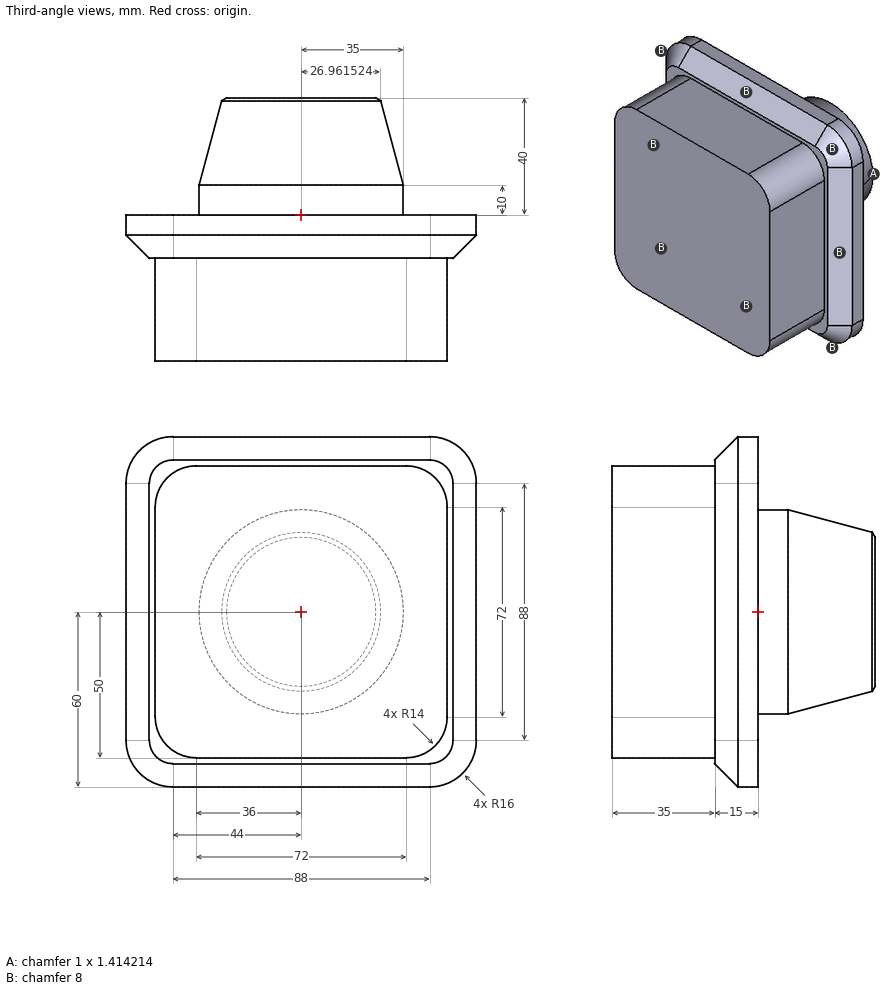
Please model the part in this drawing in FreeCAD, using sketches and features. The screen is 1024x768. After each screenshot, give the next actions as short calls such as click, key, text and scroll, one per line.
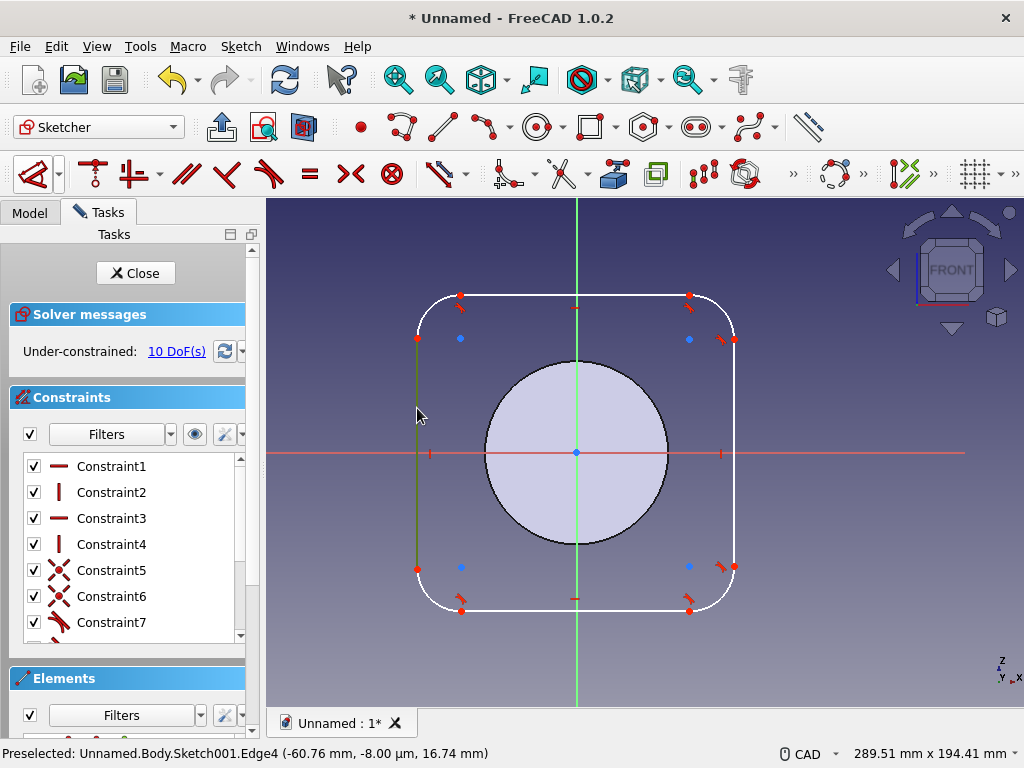
click(441, 300)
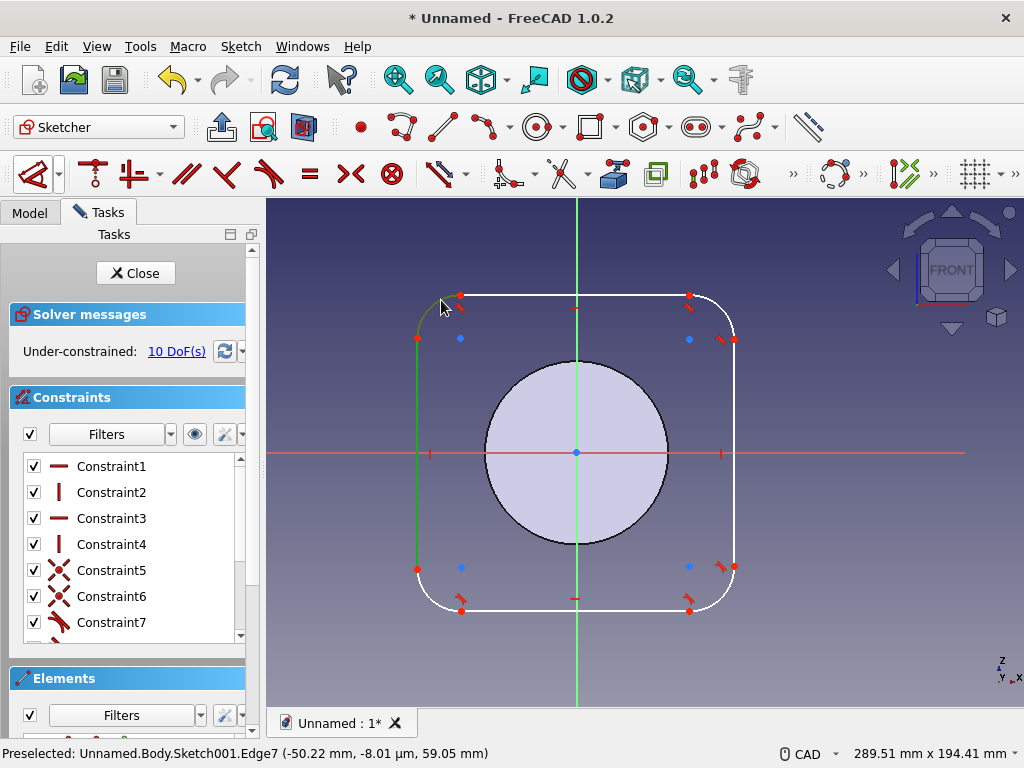
key(t)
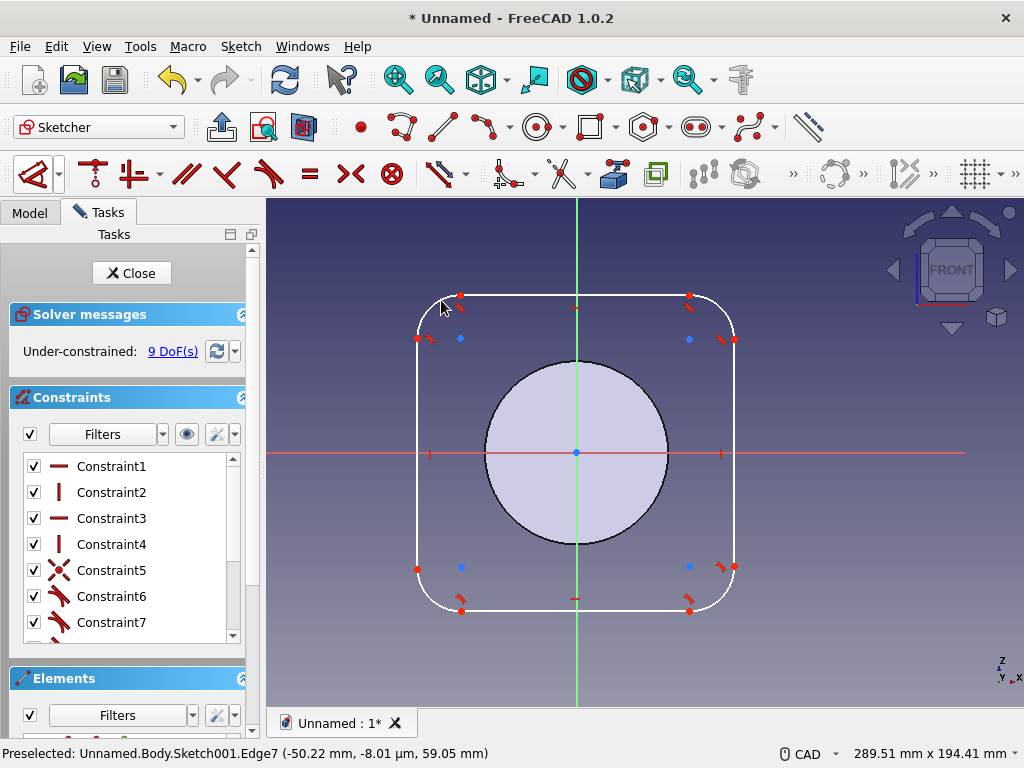
click(417, 408)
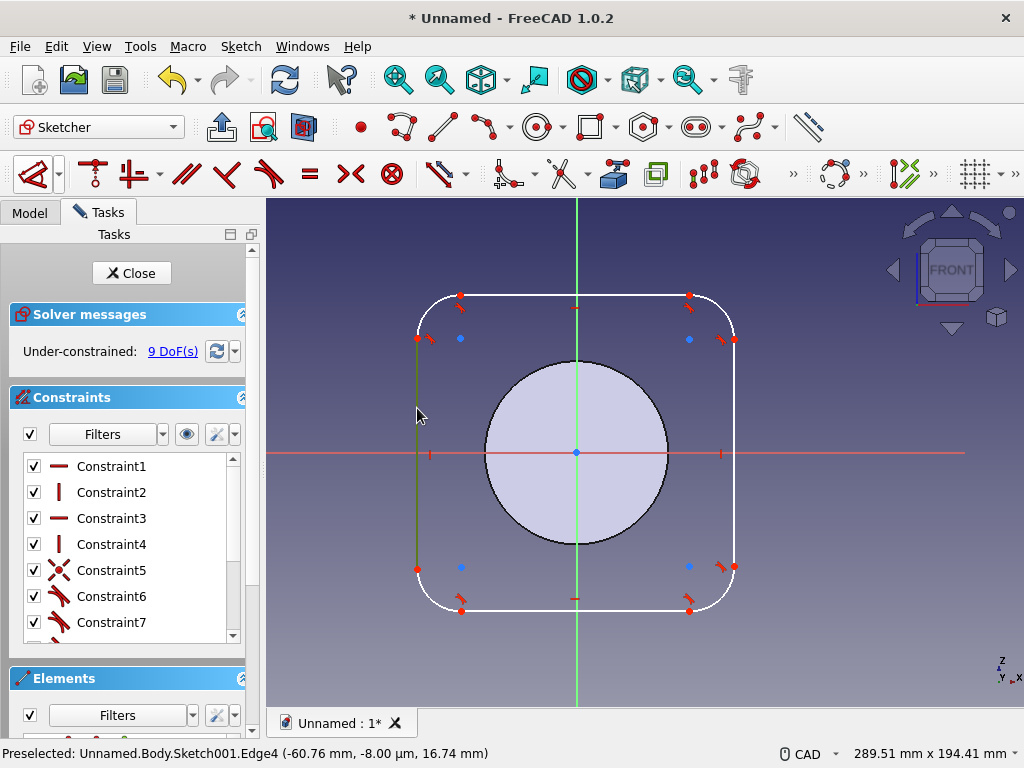
click(423, 589)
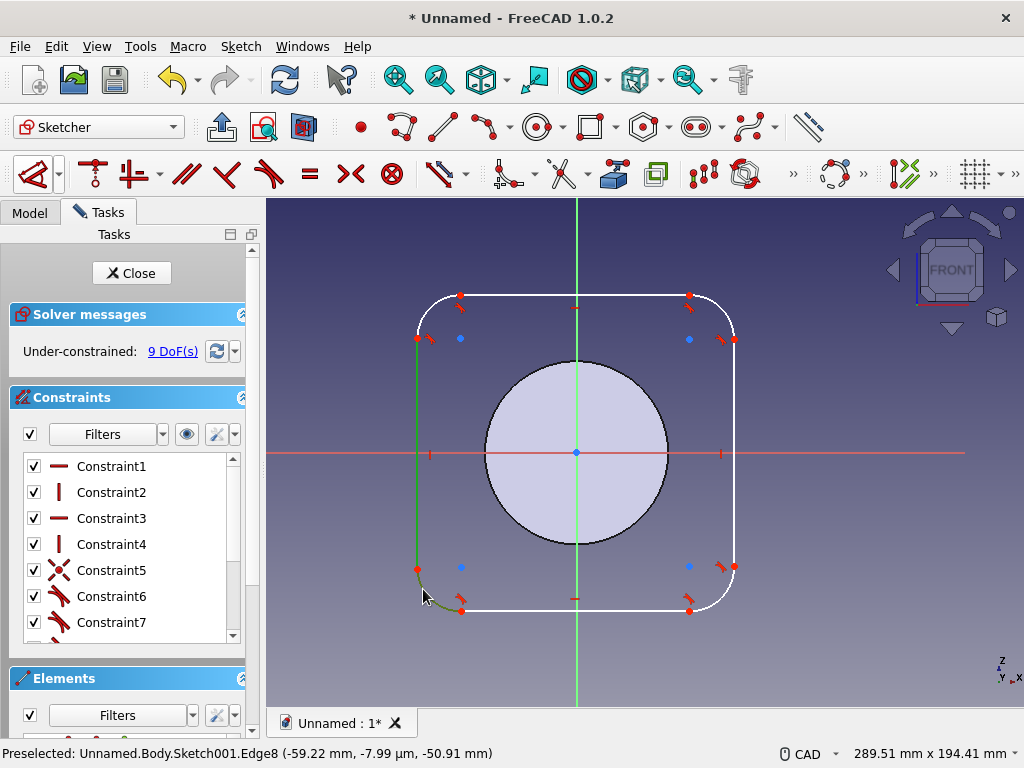
key(t)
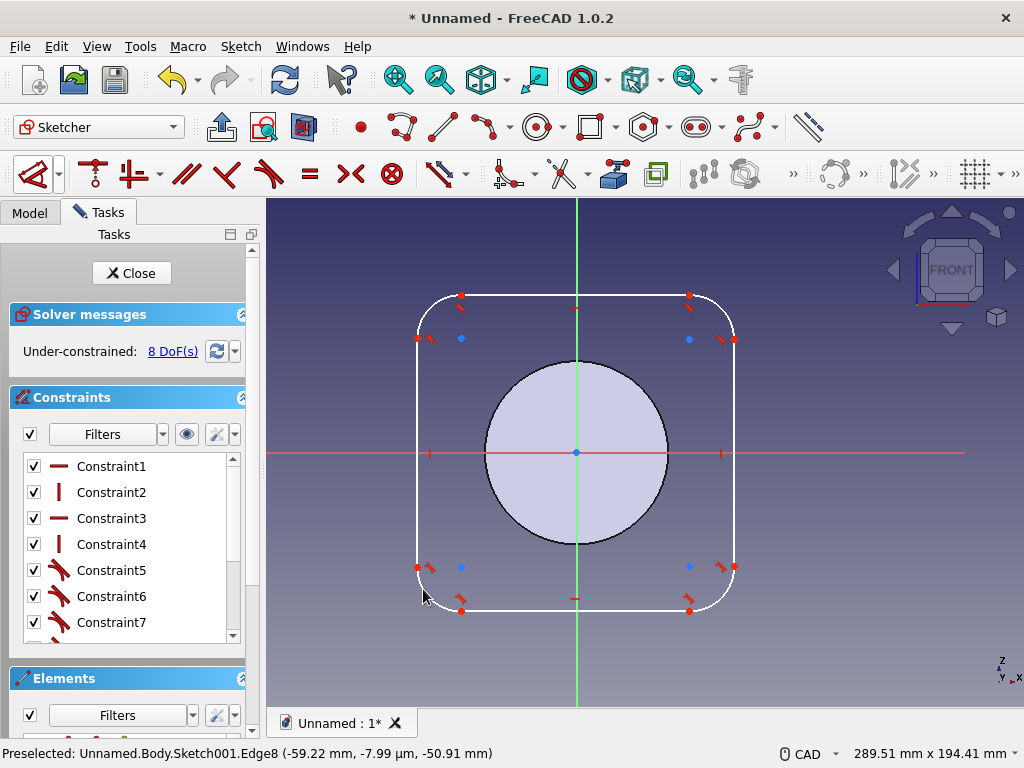
click(710, 607)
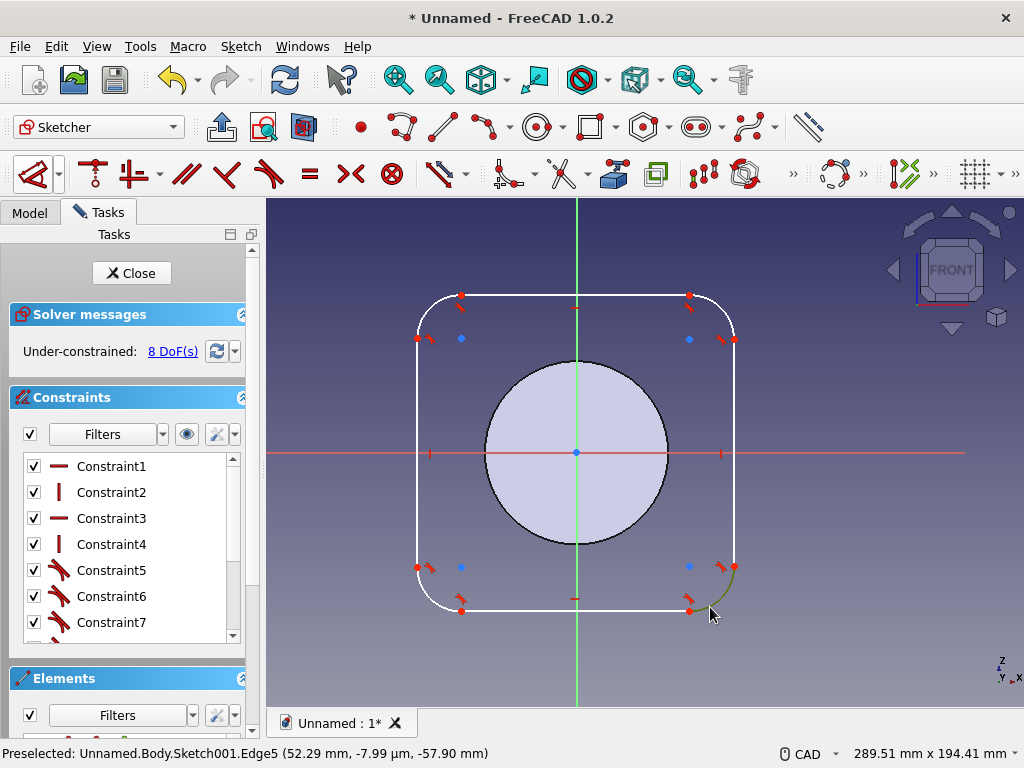
click(729, 319)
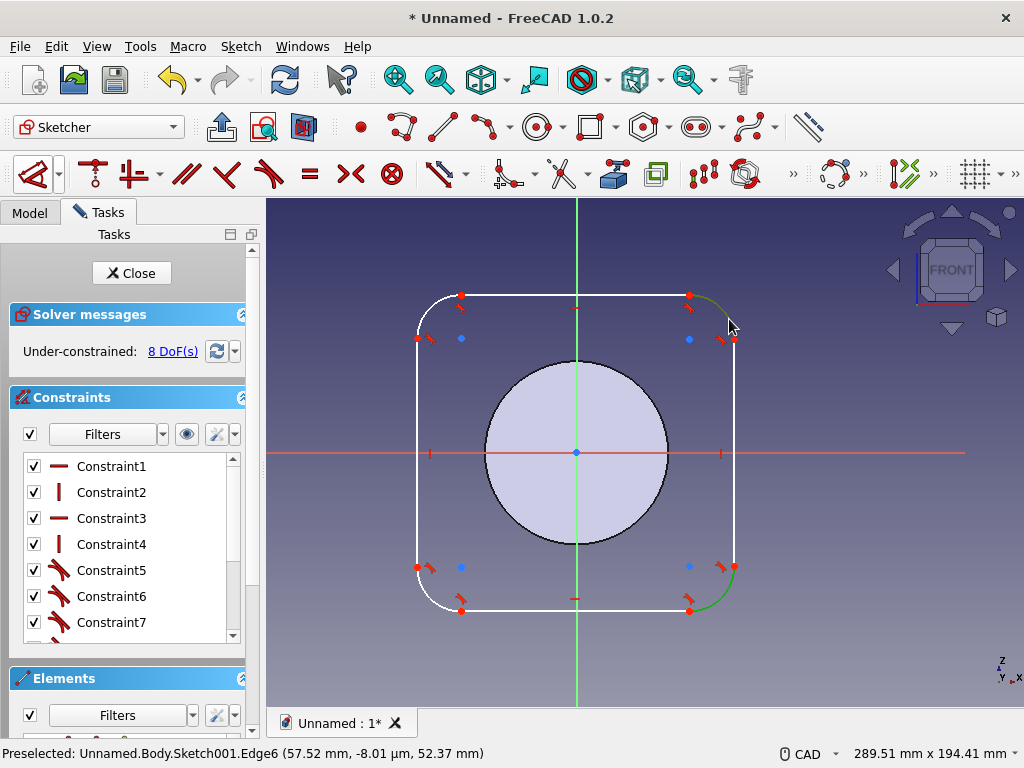
click(441, 300)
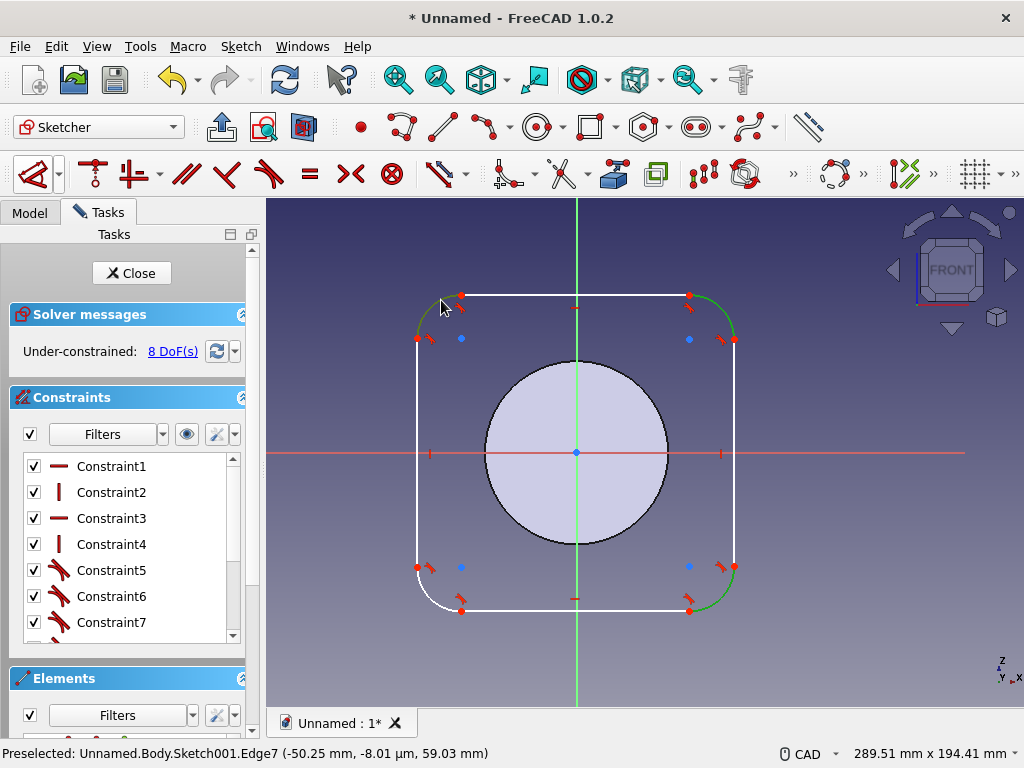
click(422, 588)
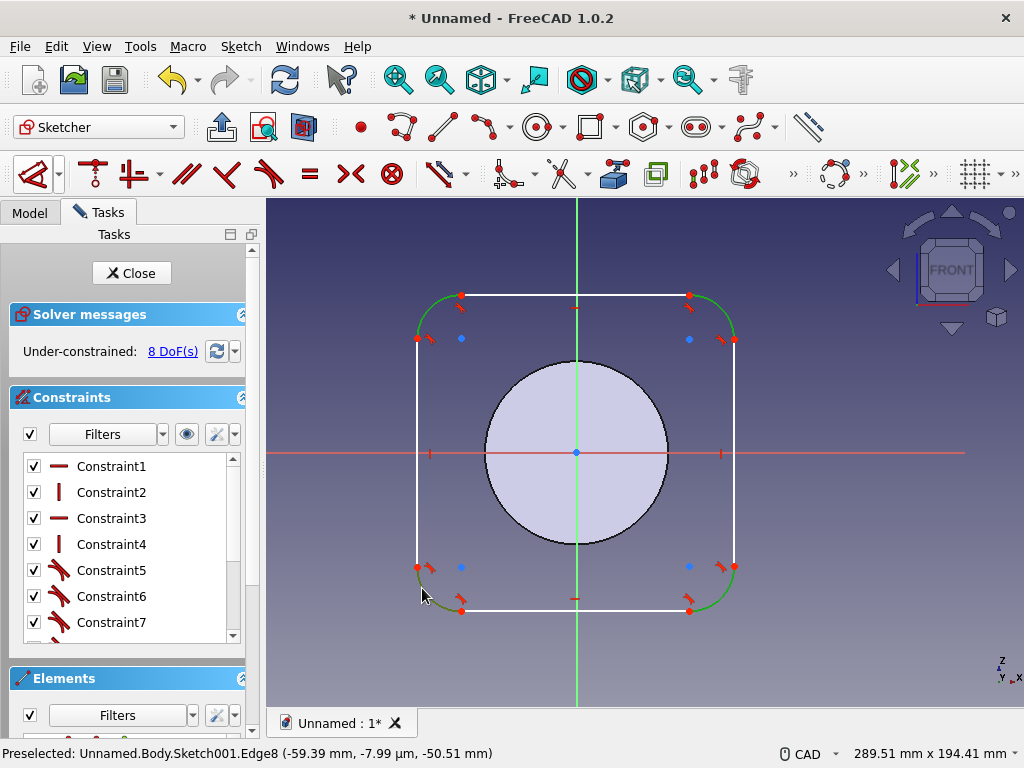
click(310, 174)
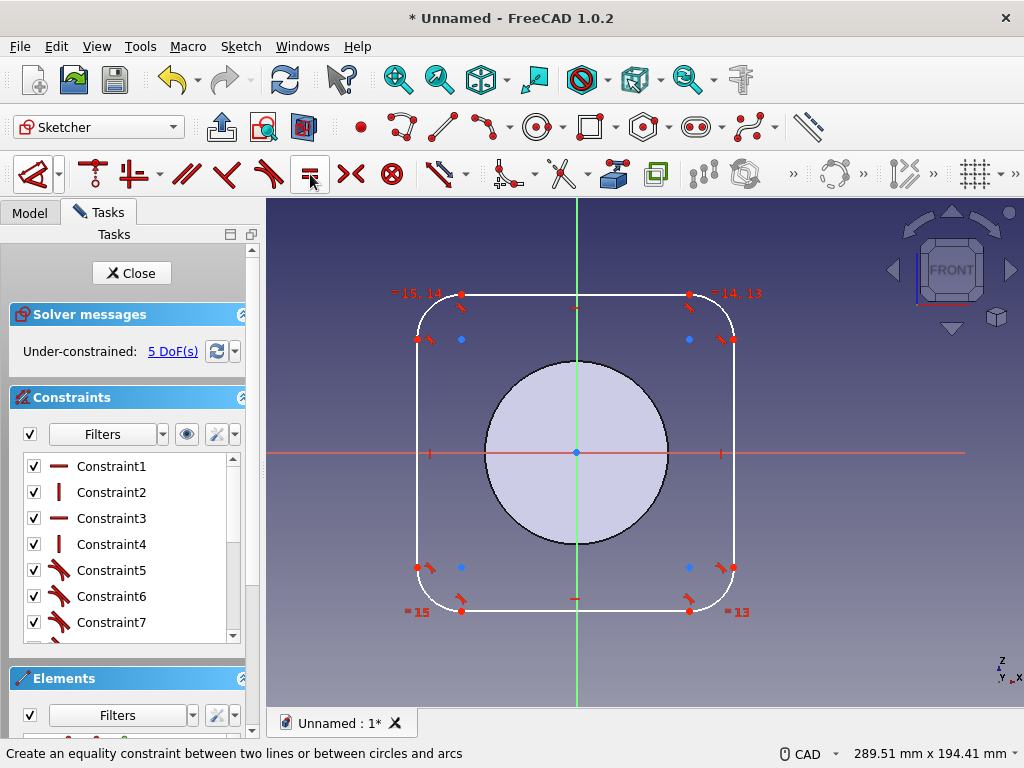
key(d)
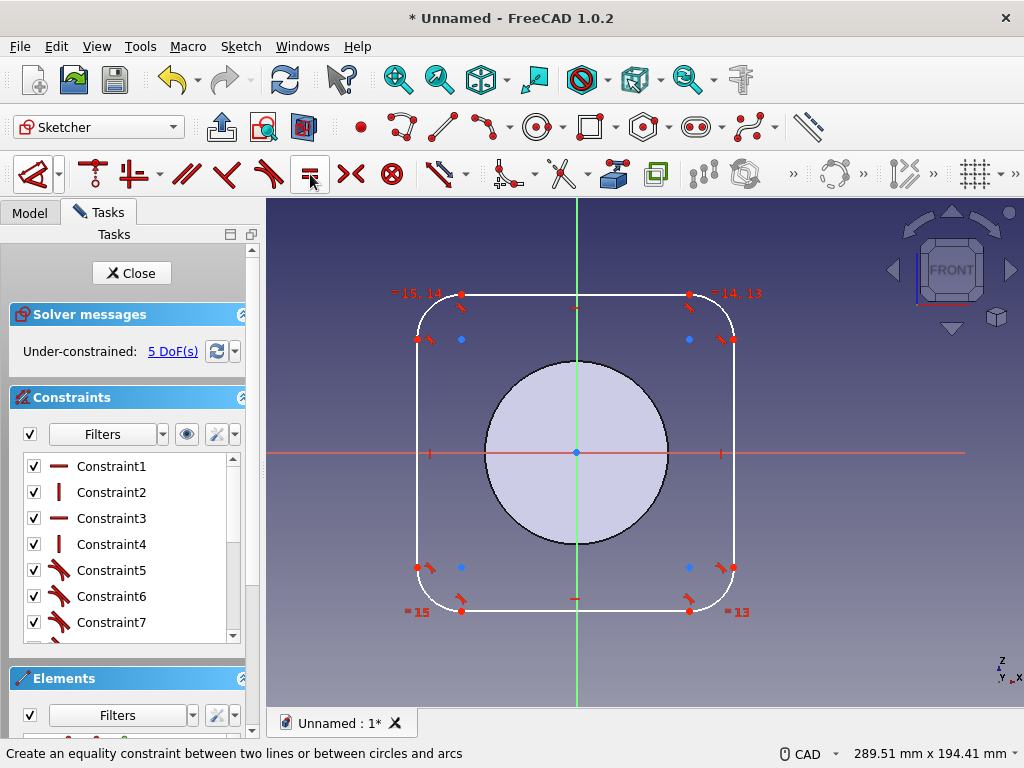
click(710, 606)
click(725, 634)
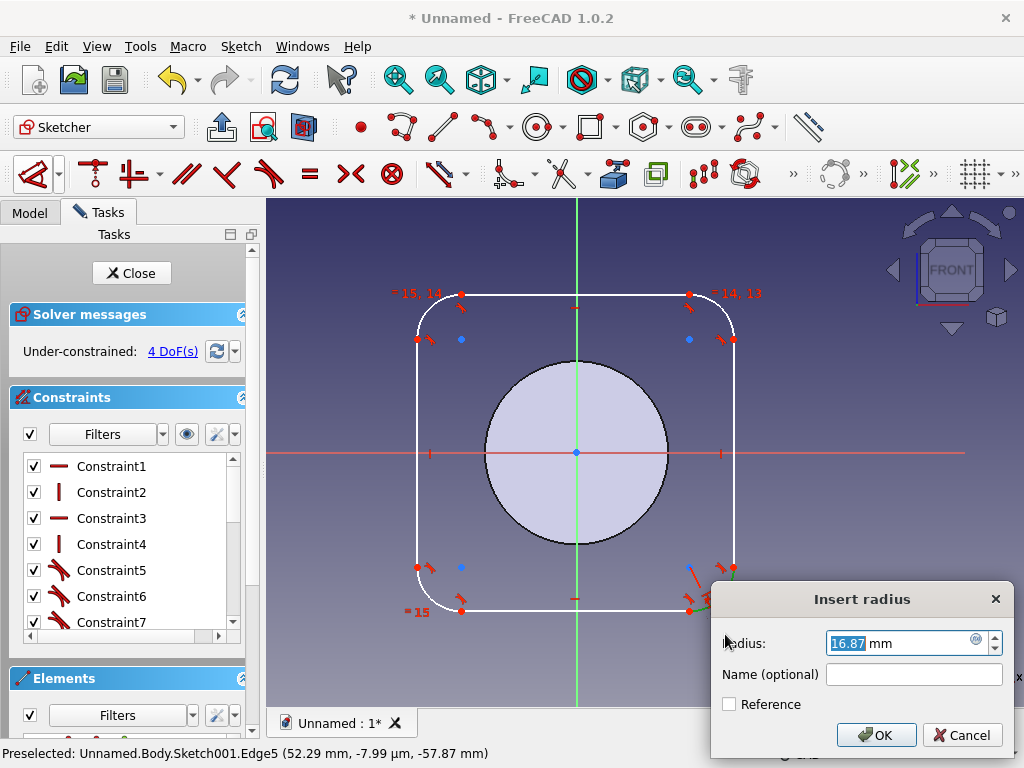
text(16)
key(Return)